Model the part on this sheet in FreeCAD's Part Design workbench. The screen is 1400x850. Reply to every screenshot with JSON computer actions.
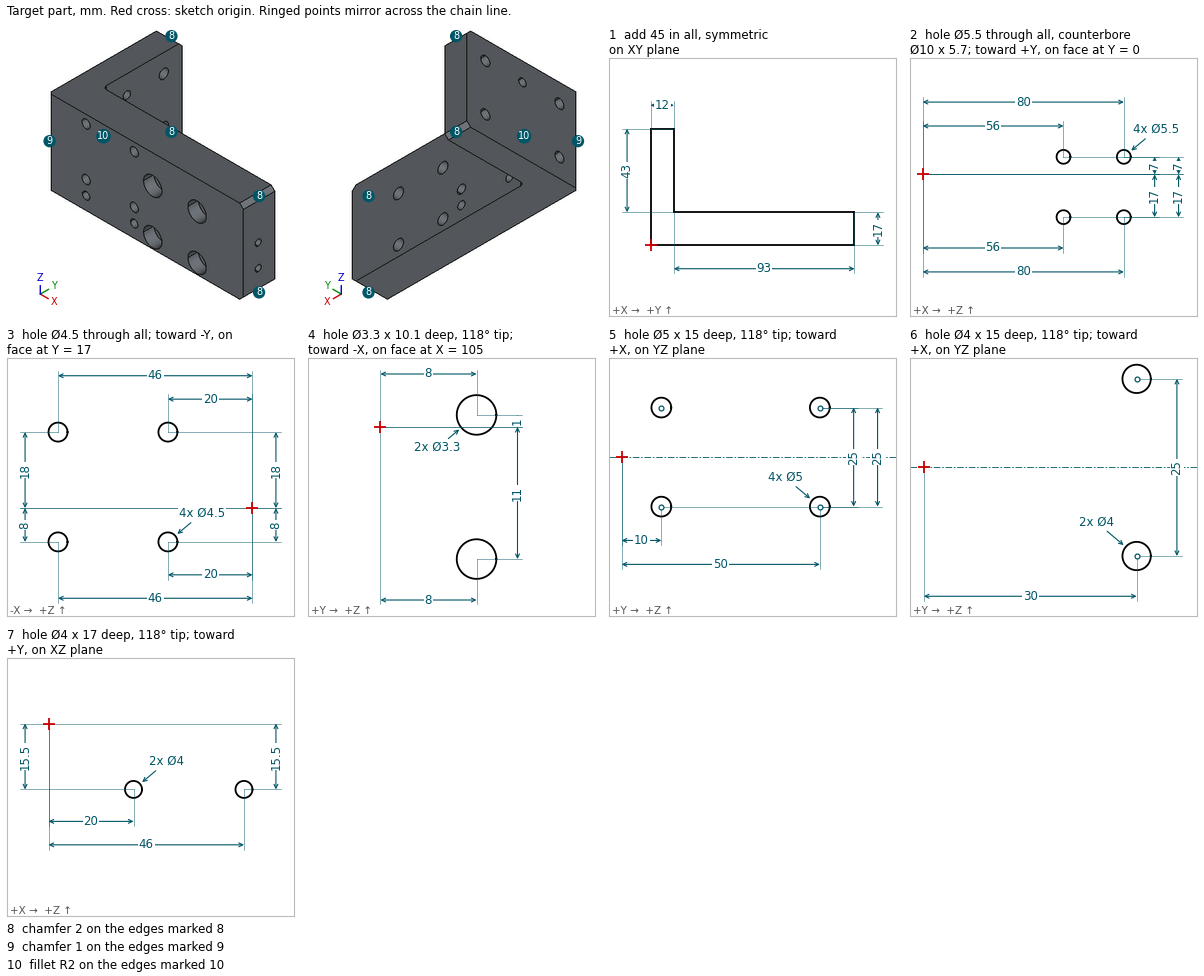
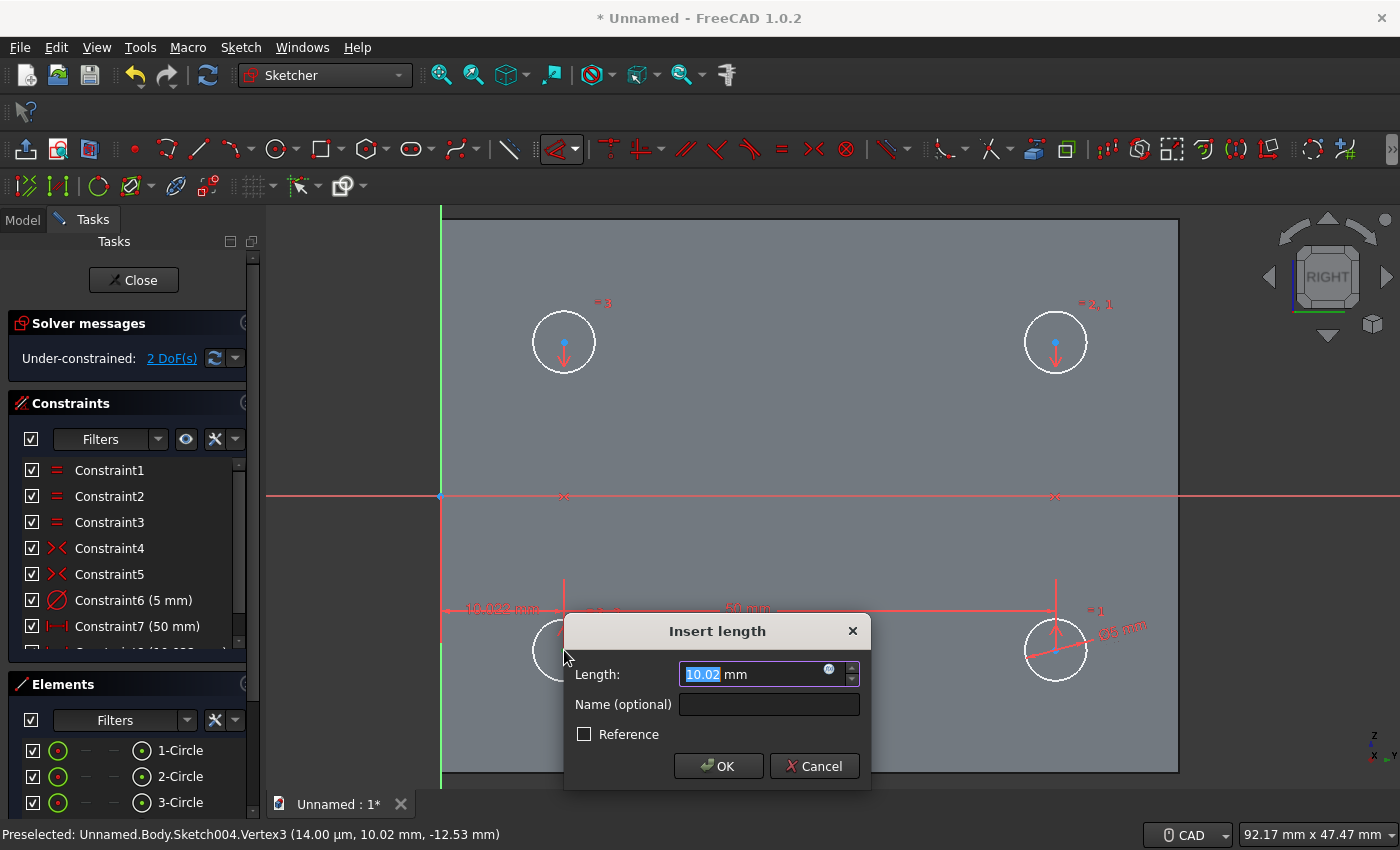
{"action": "type", "text": "10"}
{"action": "key", "text": "Return"}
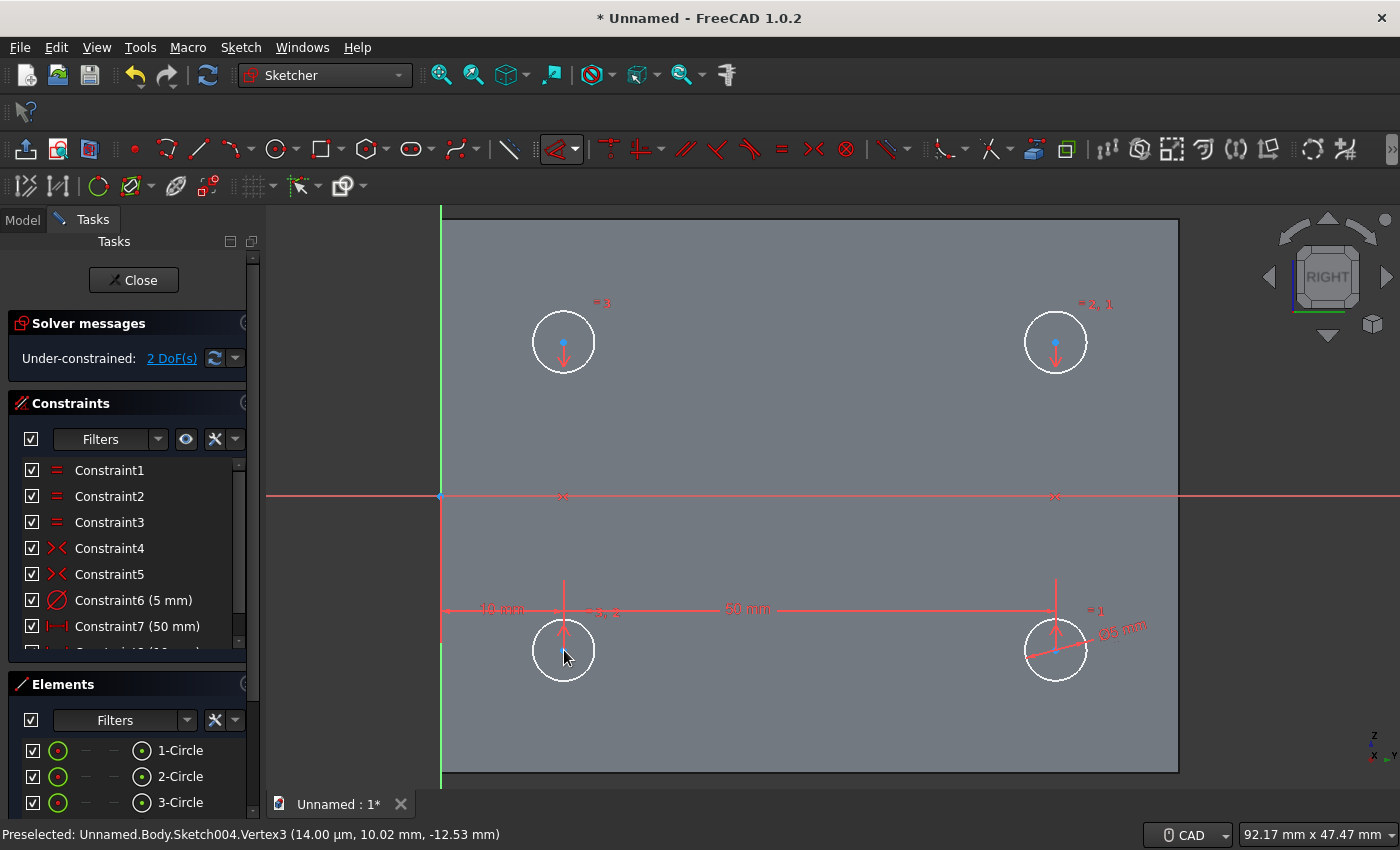
{"action": "left_click", "coordinate": [1056, 650]}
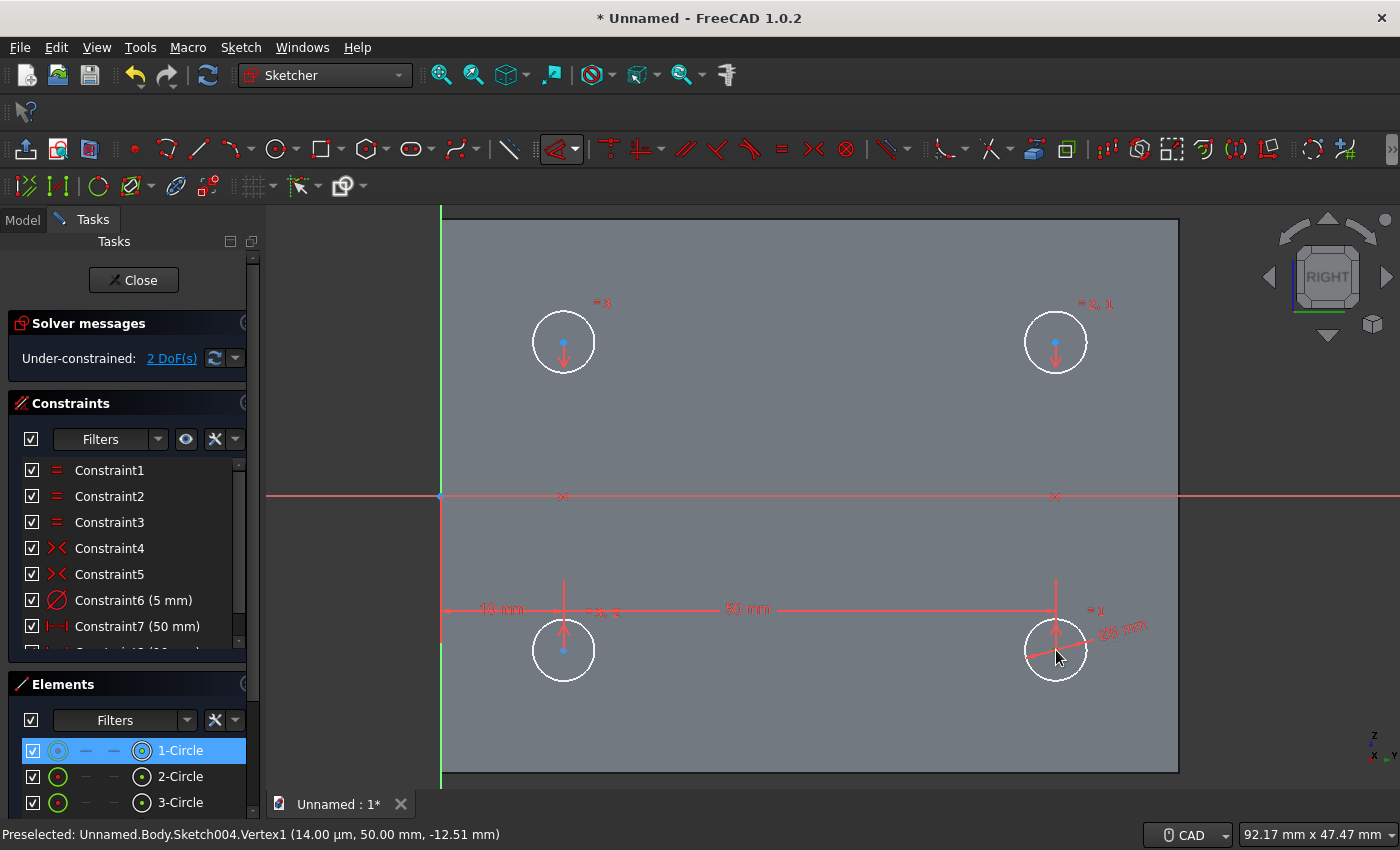
{"action": "left_click", "coordinate": [1056, 342]}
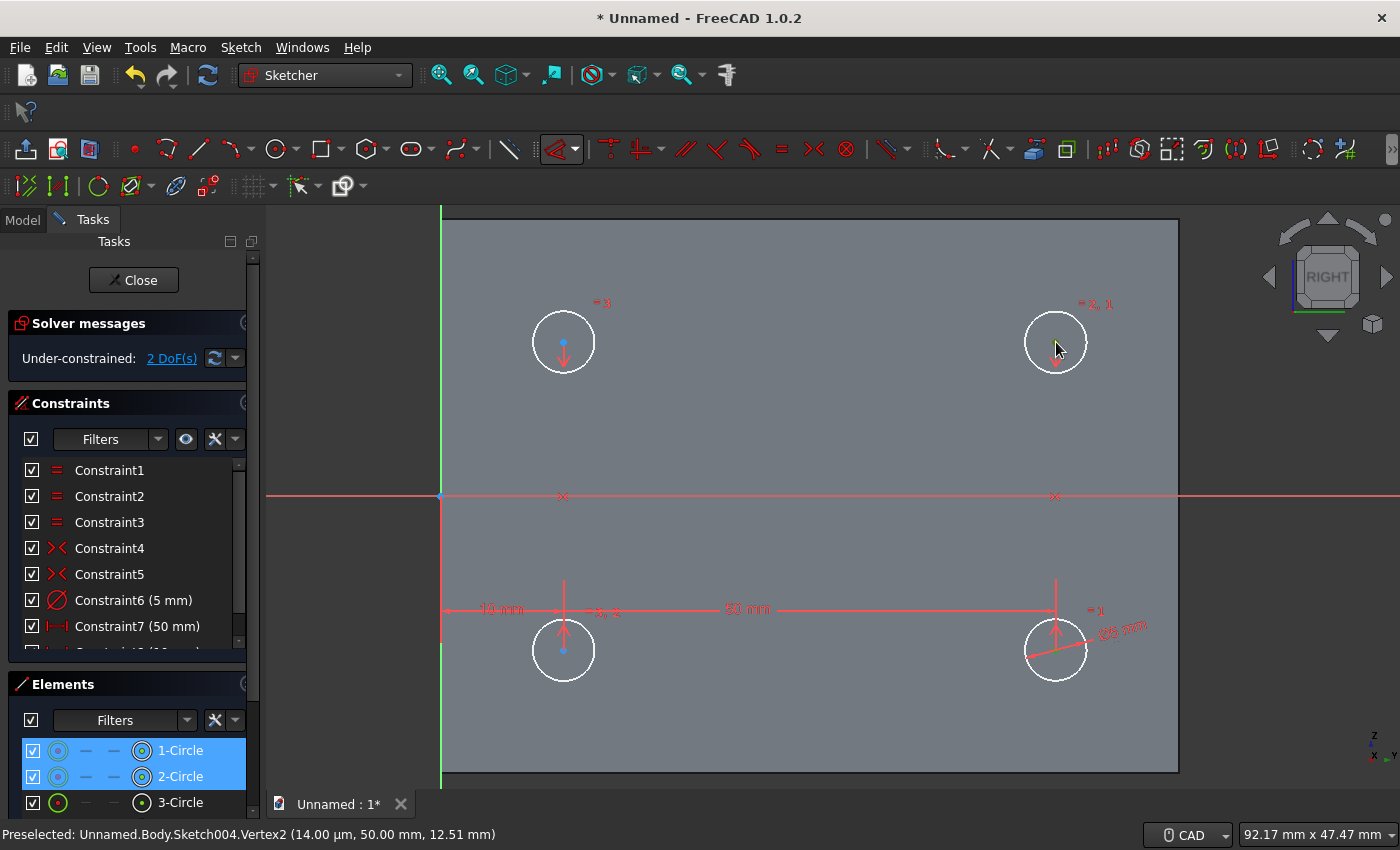
{"action": "key", "text": "i"}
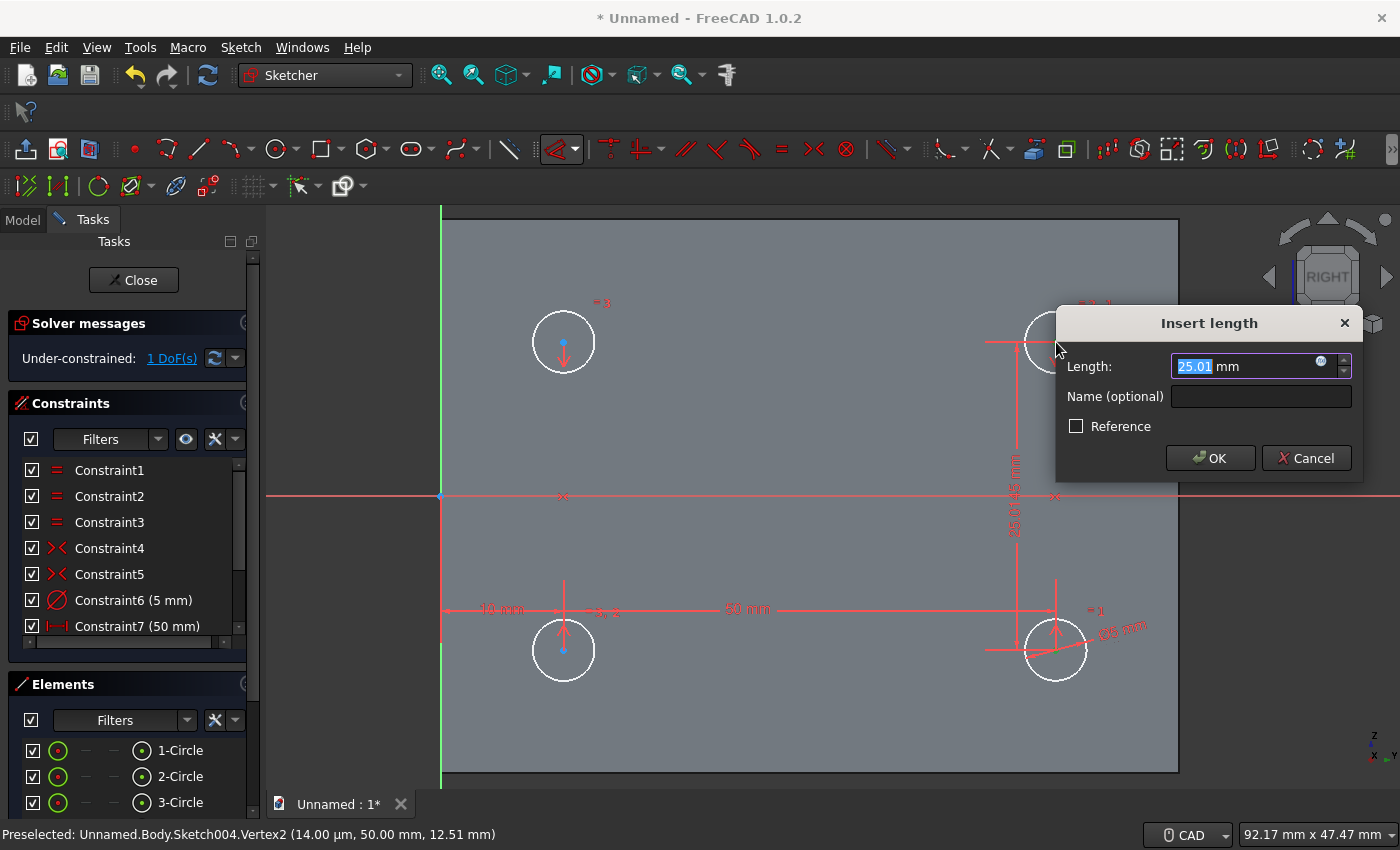
{"action": "type", "text": "25"}
{"action": "key", "text": "Return"}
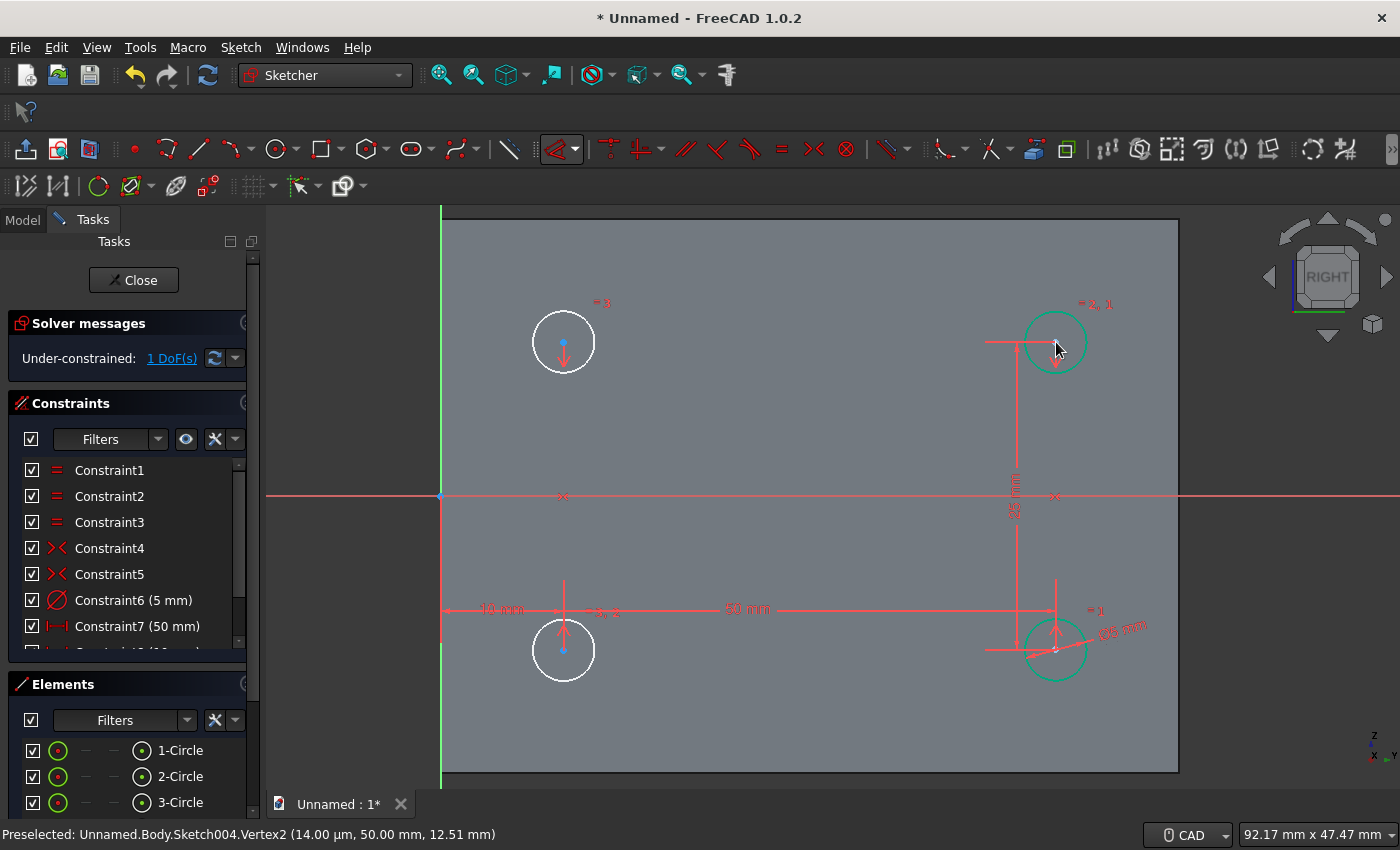
{"action": "left_click", "coordinate": [1056, 342]}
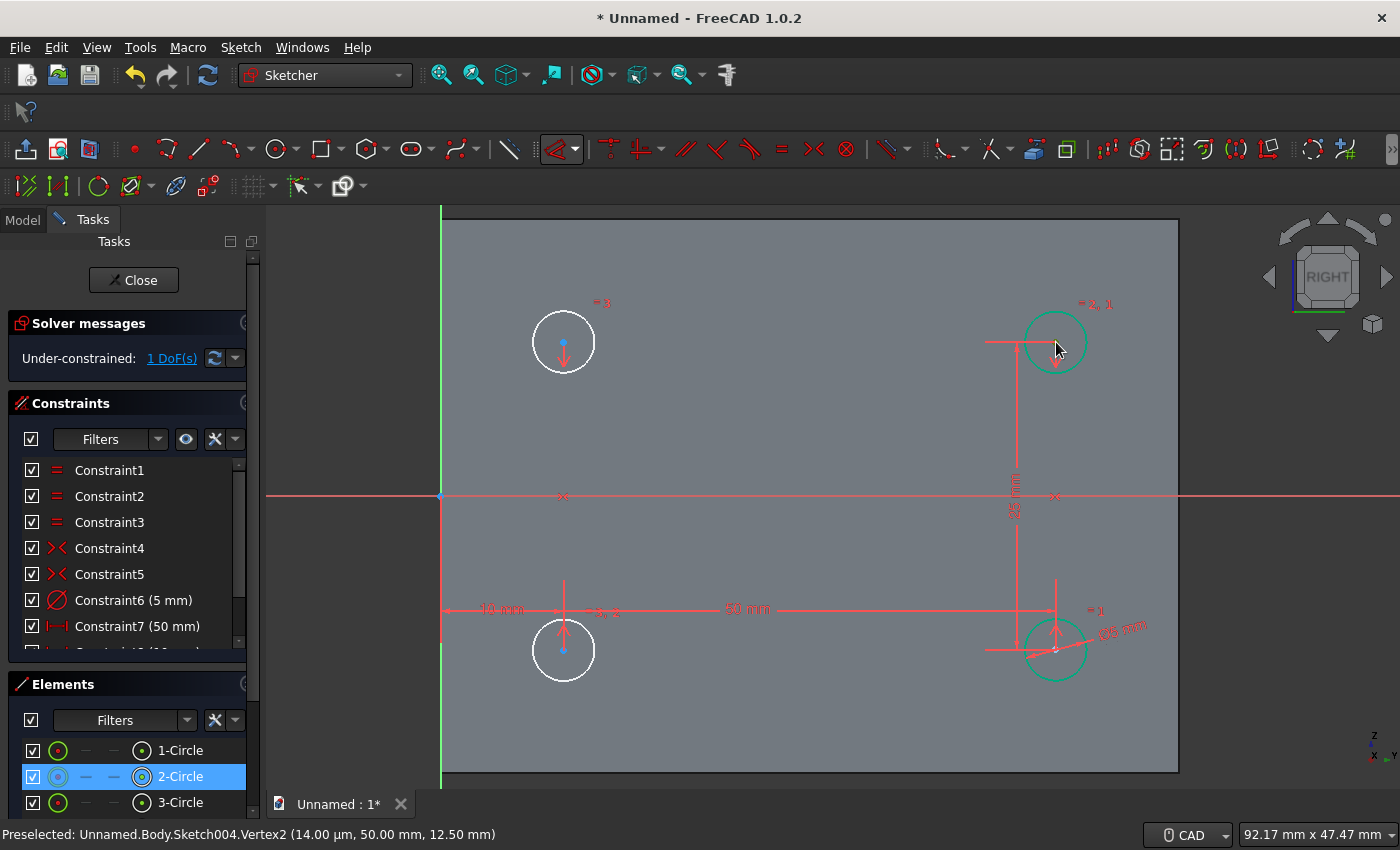
{"action": "left_click", "coordinate": [564, 650]}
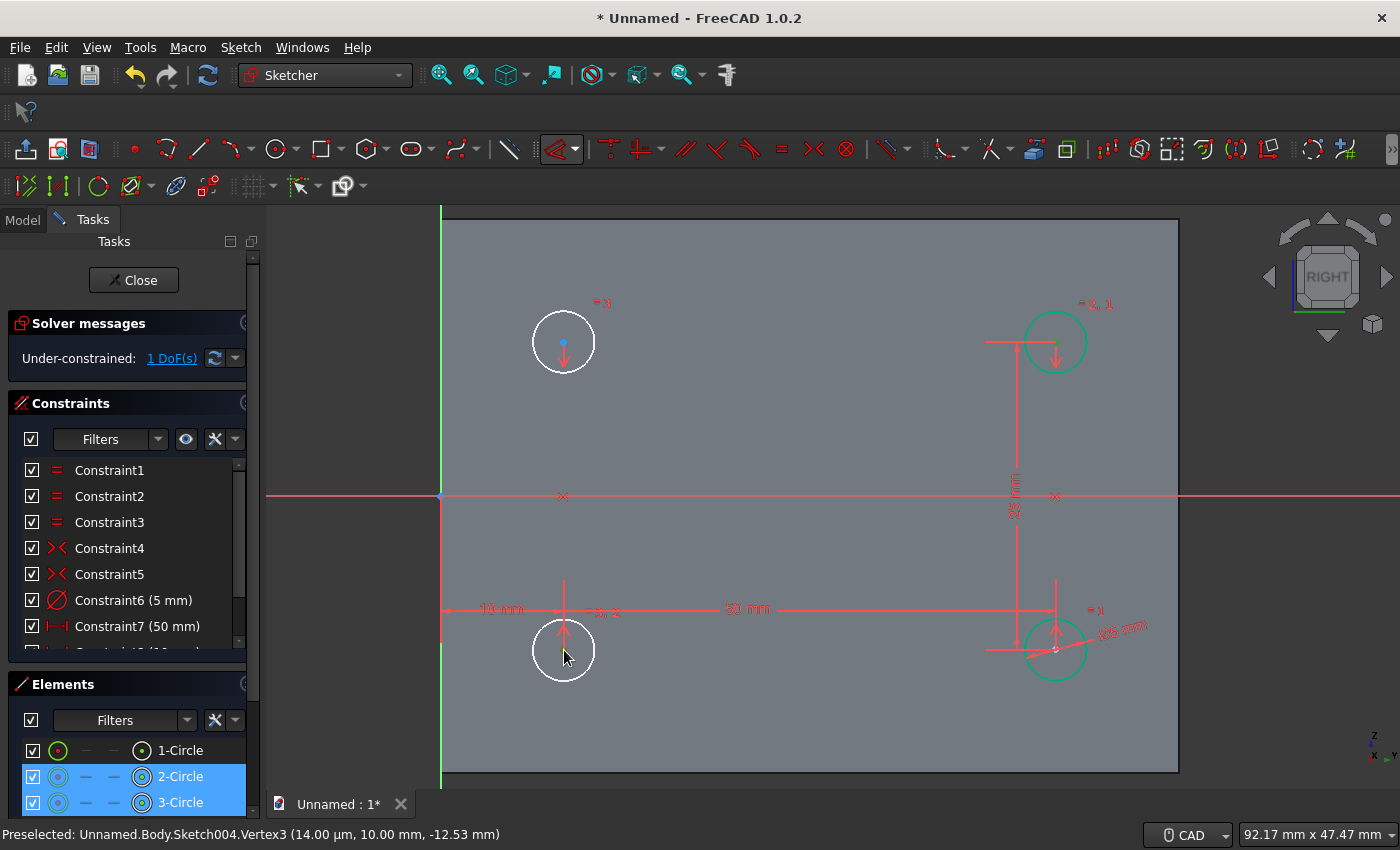
{"action": "key", "text": "i"}